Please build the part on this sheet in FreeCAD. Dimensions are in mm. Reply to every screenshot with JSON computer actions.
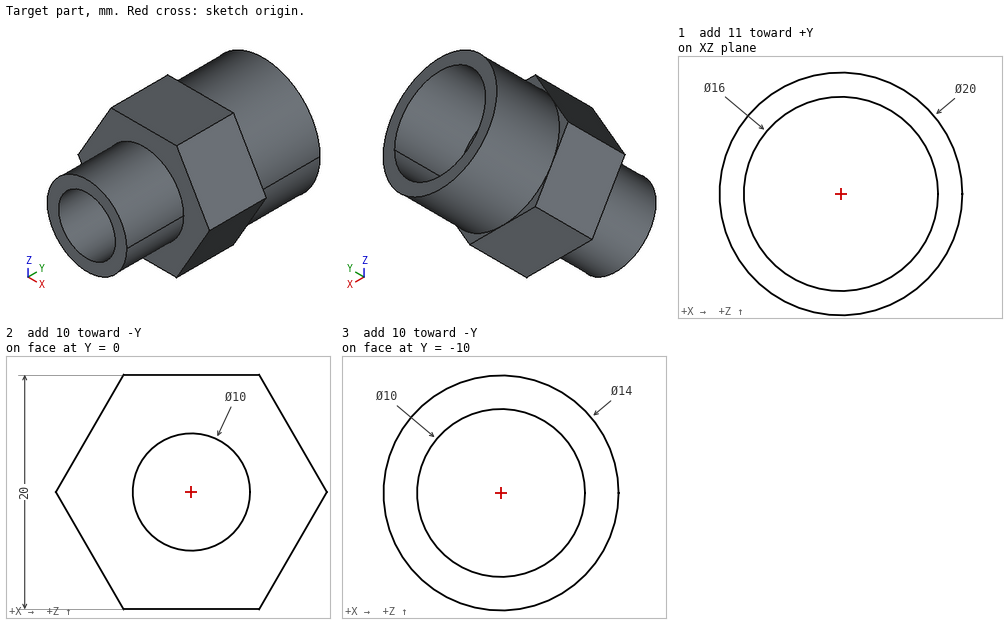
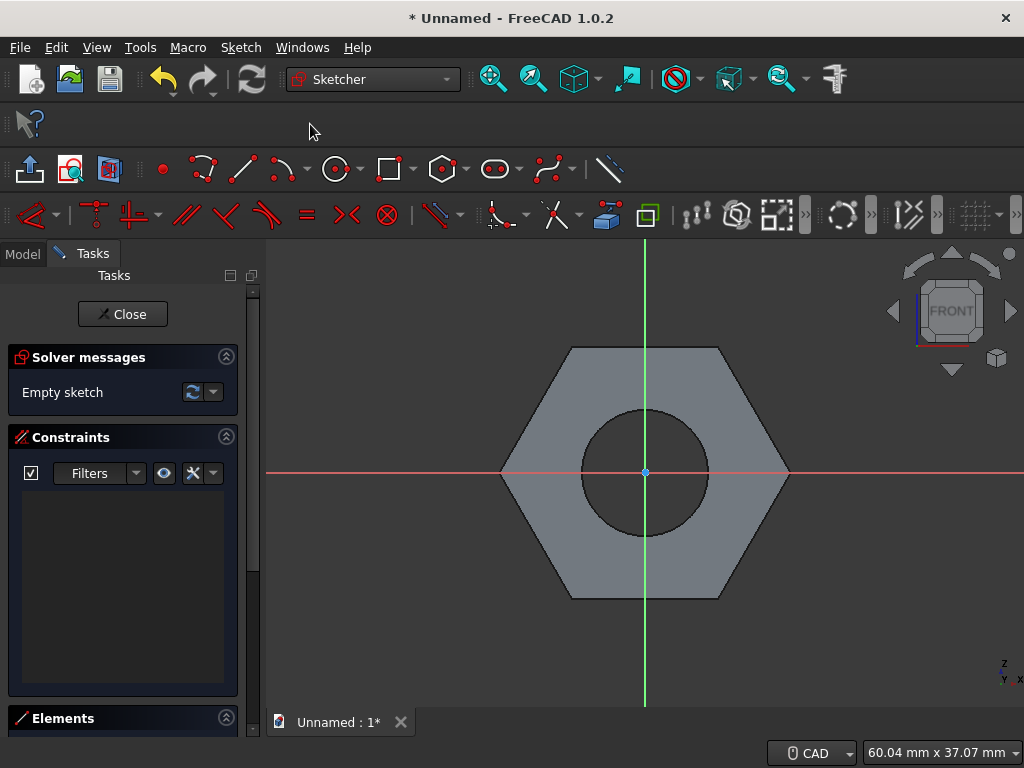
{"action": "scroll", "coordinate": [784, 473], "scroll_direction": "up", "scroll_amount": 2}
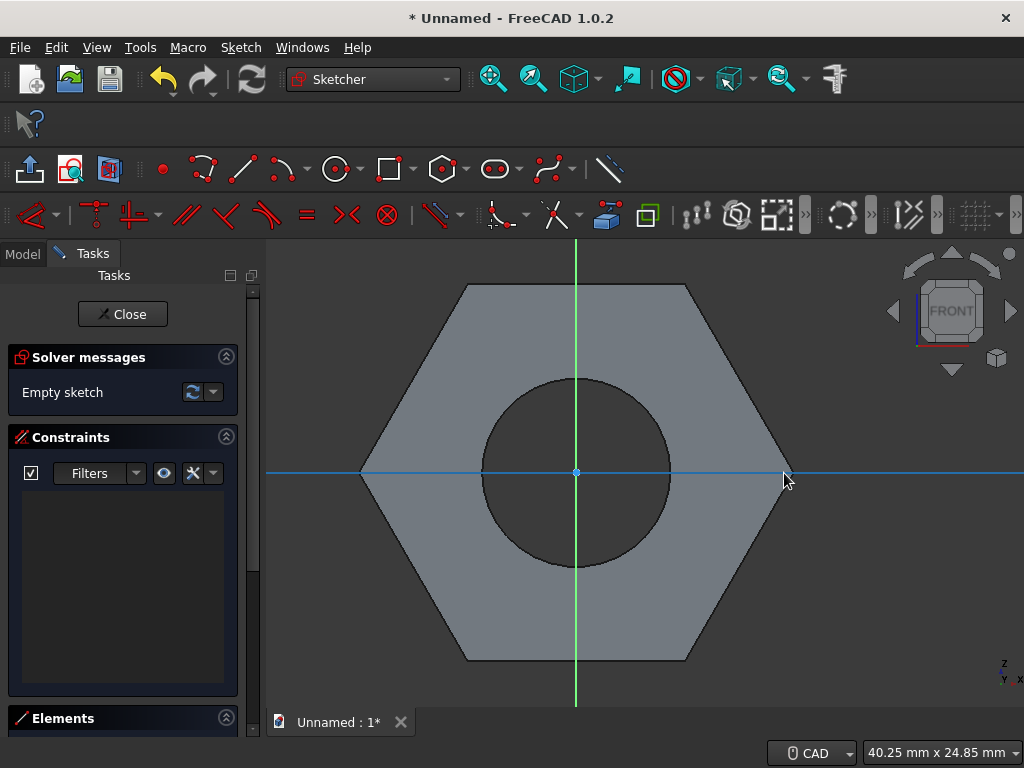
{"action": "left_click", "coordinate": [336, 170]}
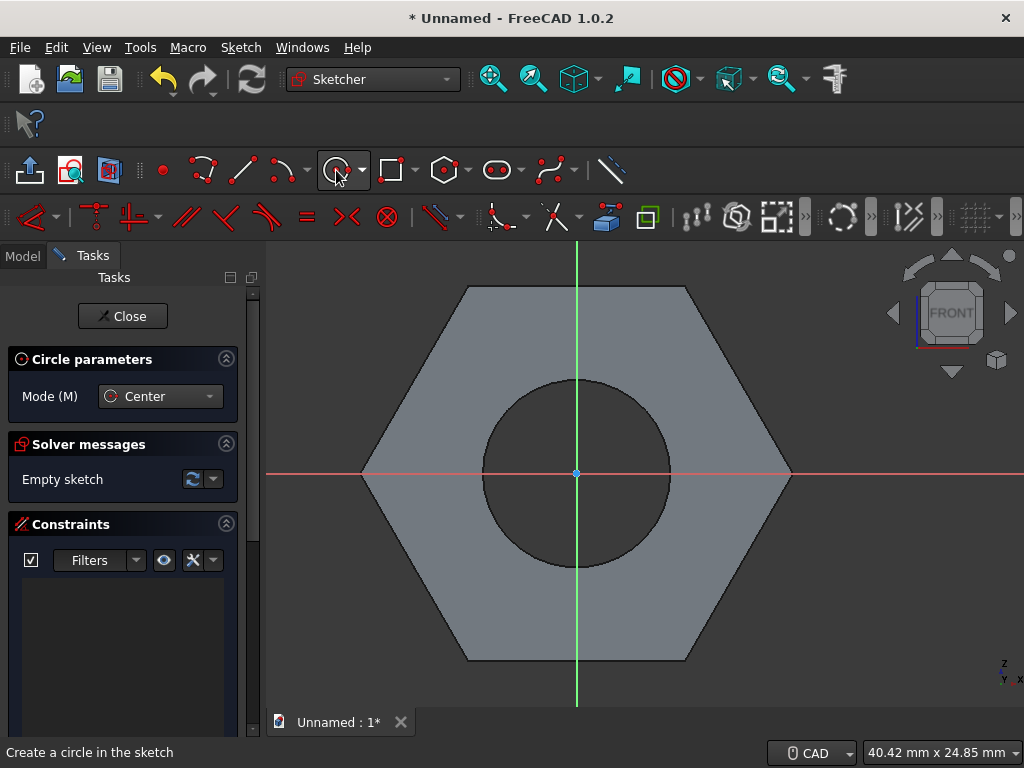
{"action": "left_click", "coordinate": [577, 474]}
{"action": "left_click", "coordinate": [669, 381]}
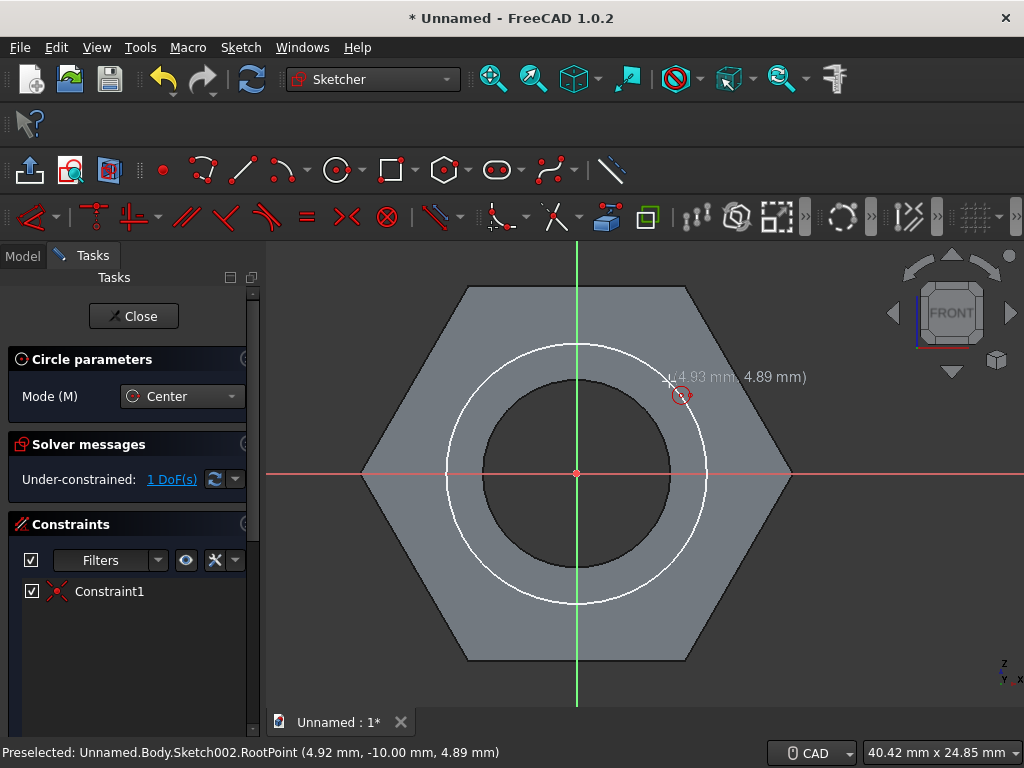
{"action": "left_click", "coordinate": [577, 474]}
{"action": "left_click", "coordinate": [643, 407]}
{"action": "key", "text": "Escape"}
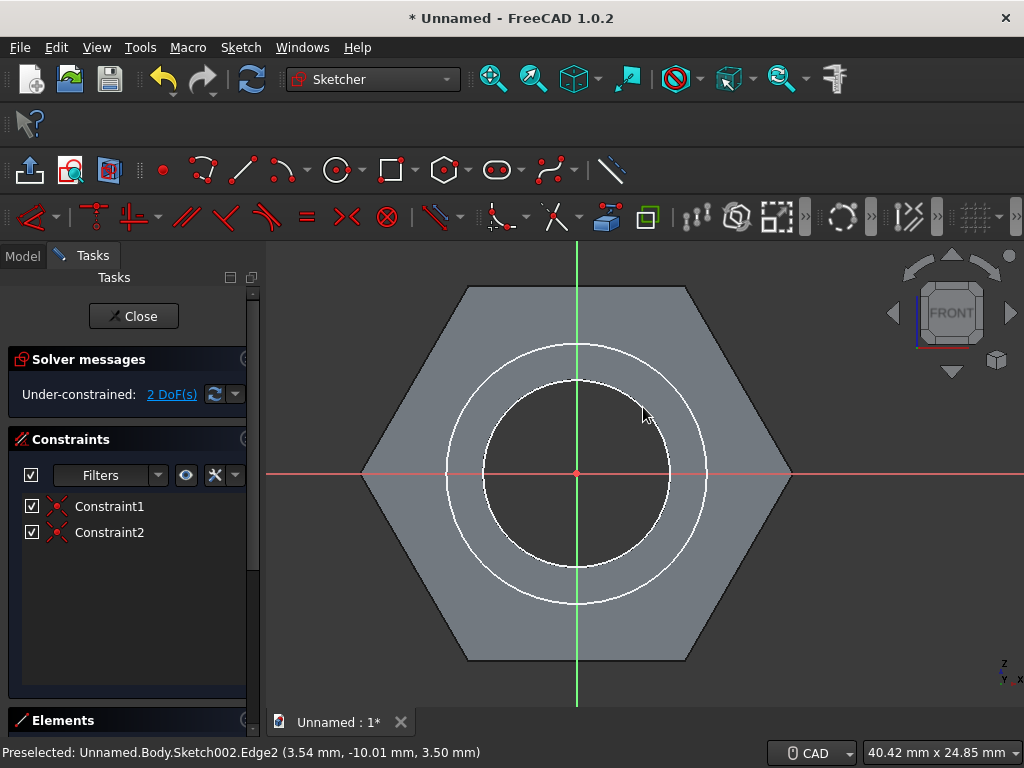
{"action": "left_click", "coordinate": [32, 218]}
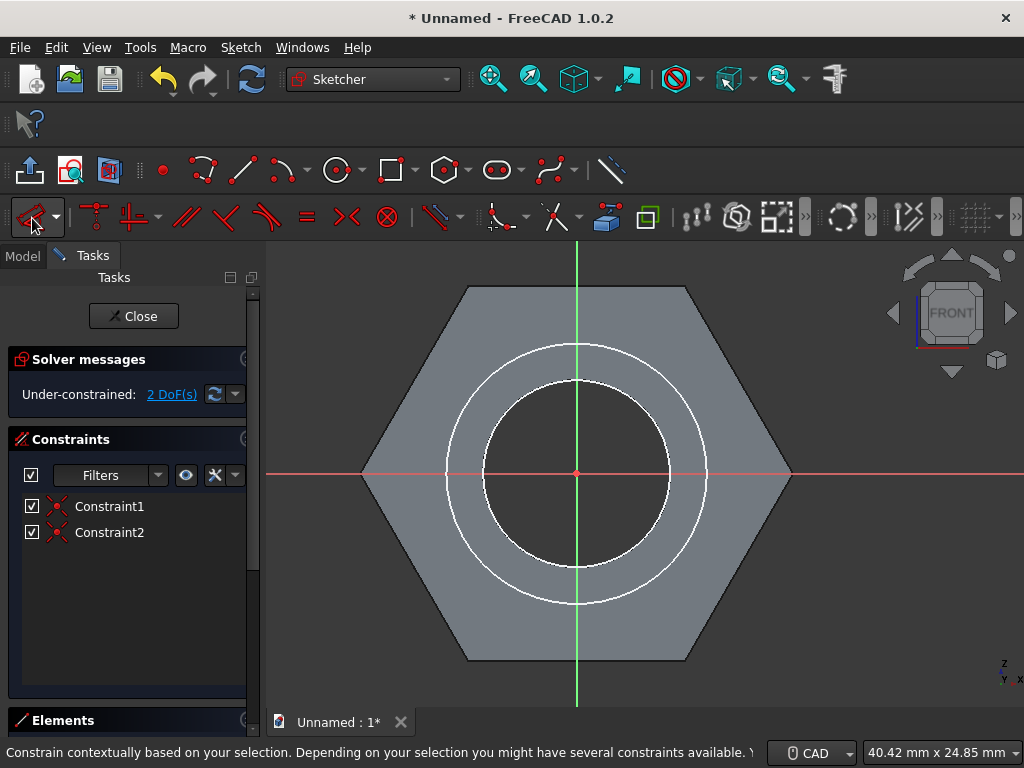
{"action": "left_click", "coordinate": [668, 381]}
{"action": "left_click", "coordinate": [690, 358]}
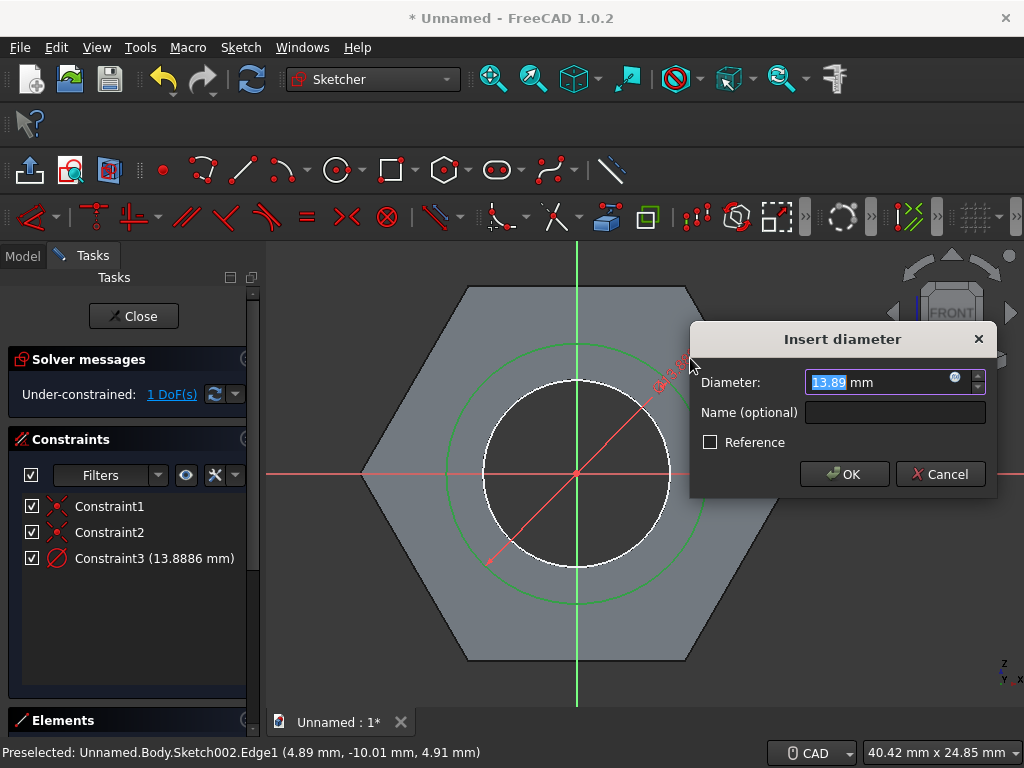
{"action": "type", "text": "14"}
{"action": "key", "text": "Return"}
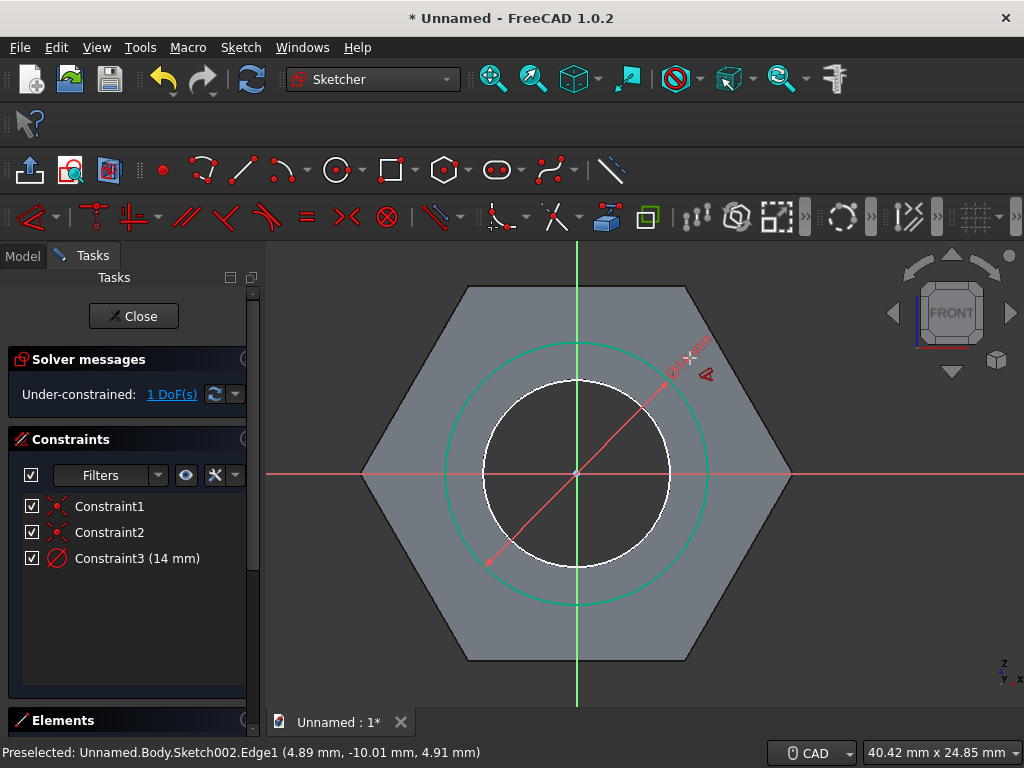
{"action": "left_click", "coordinate": [642, 407]}
{"action": "left_click", "coordinate": [719, 431]}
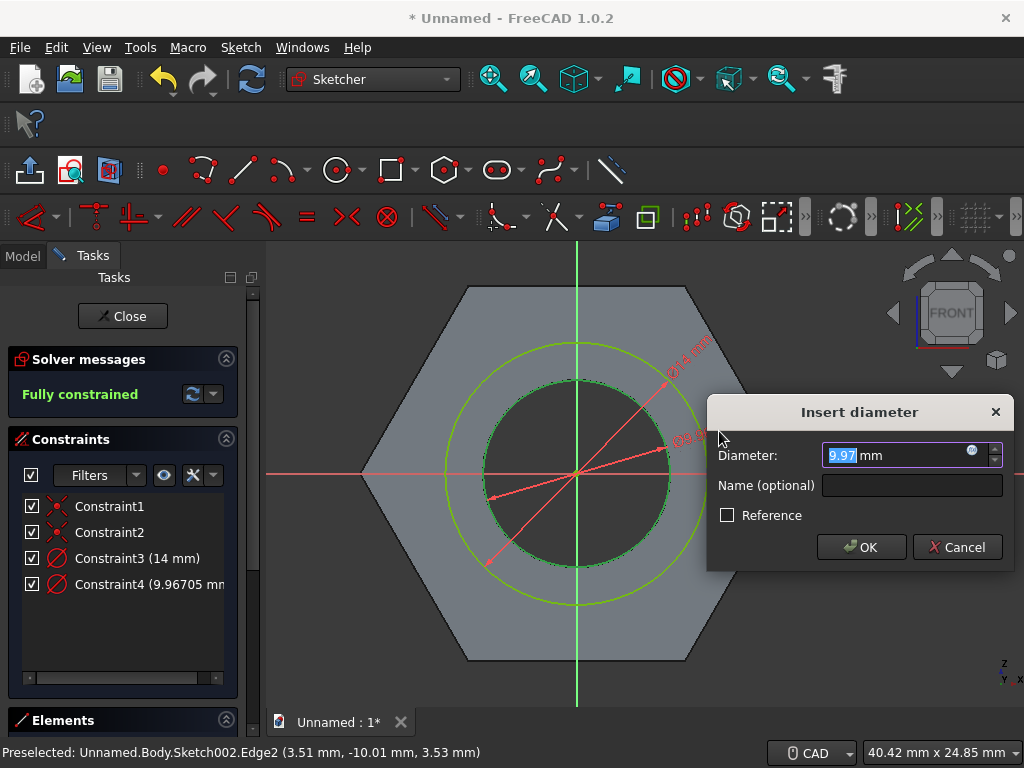
{"action": "type", "text": "10"}
{"action": "key", "text": "Return"}
{"action": "key", "text": "Escape"}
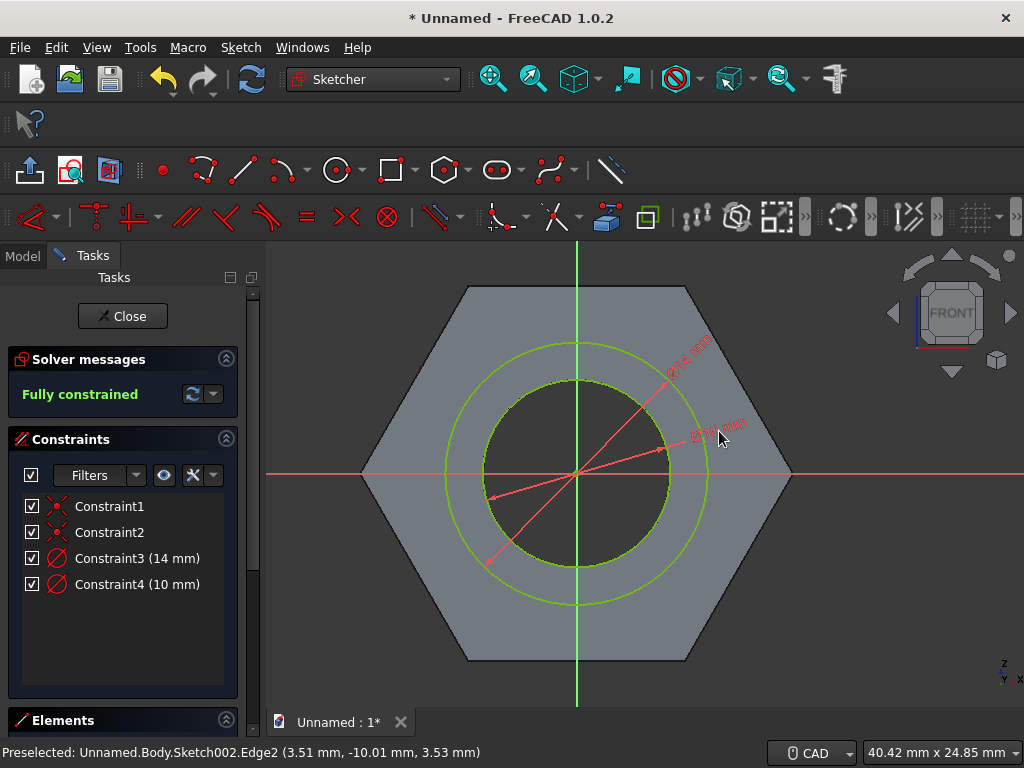
{"action": "left_click", "coordinate": [123, 316]}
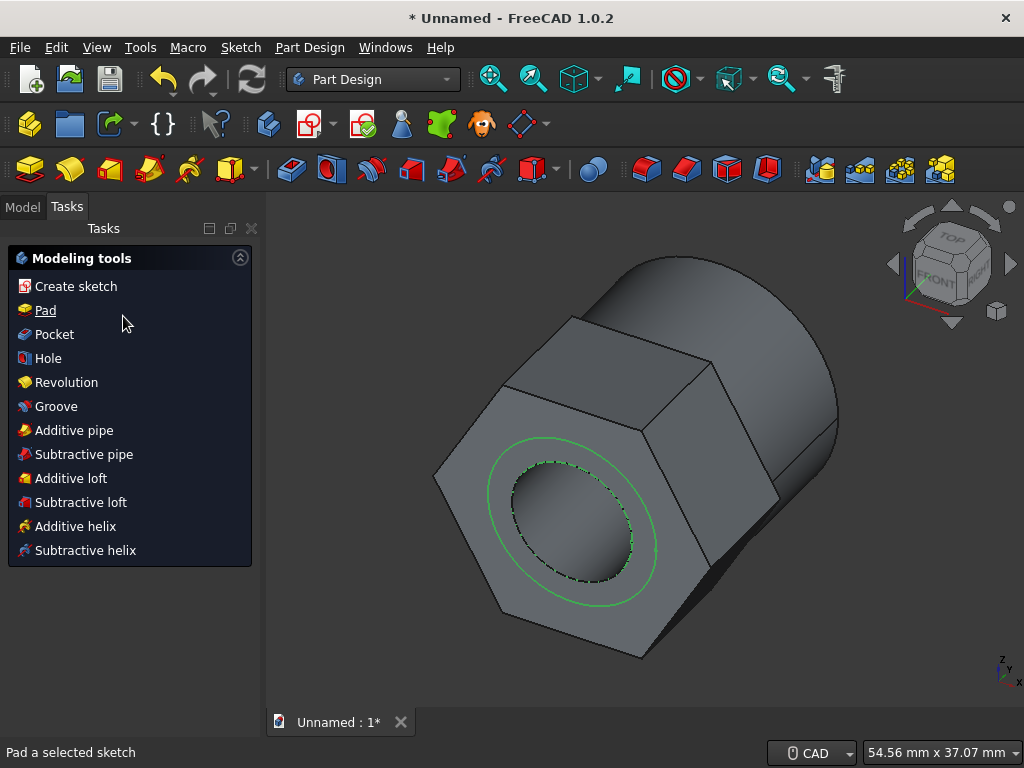
{"action": "left_click", "coordinate": [30, 170]}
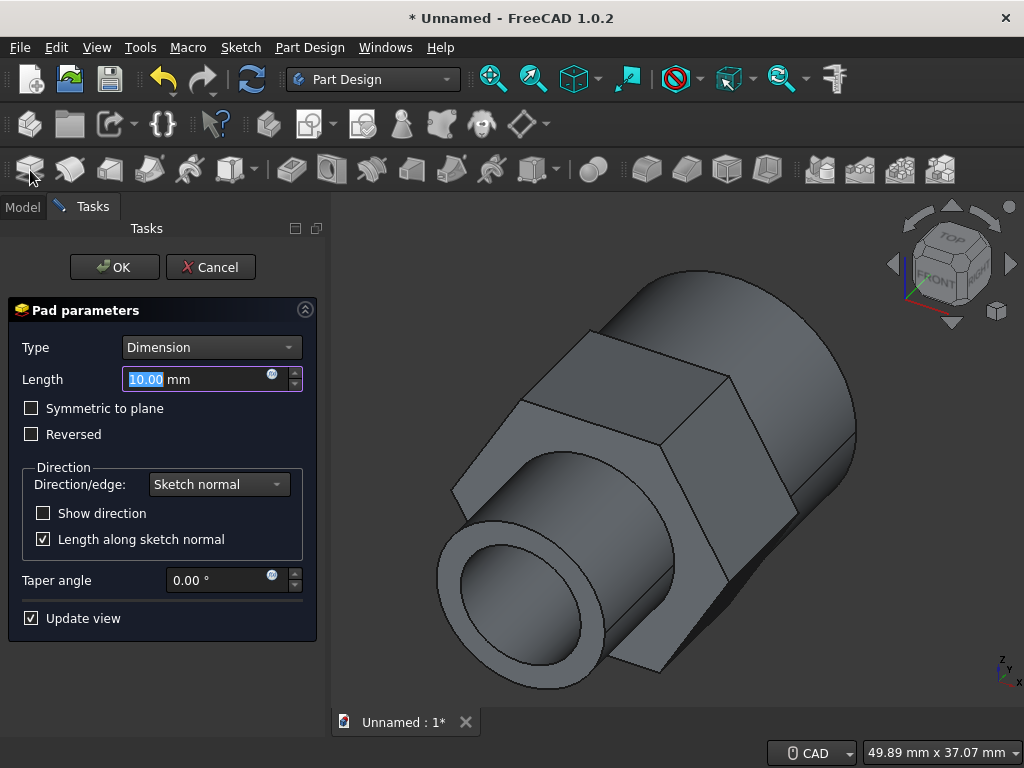
{"action": "type", "text": "10"}
{"action": "key", "text": "Tab"}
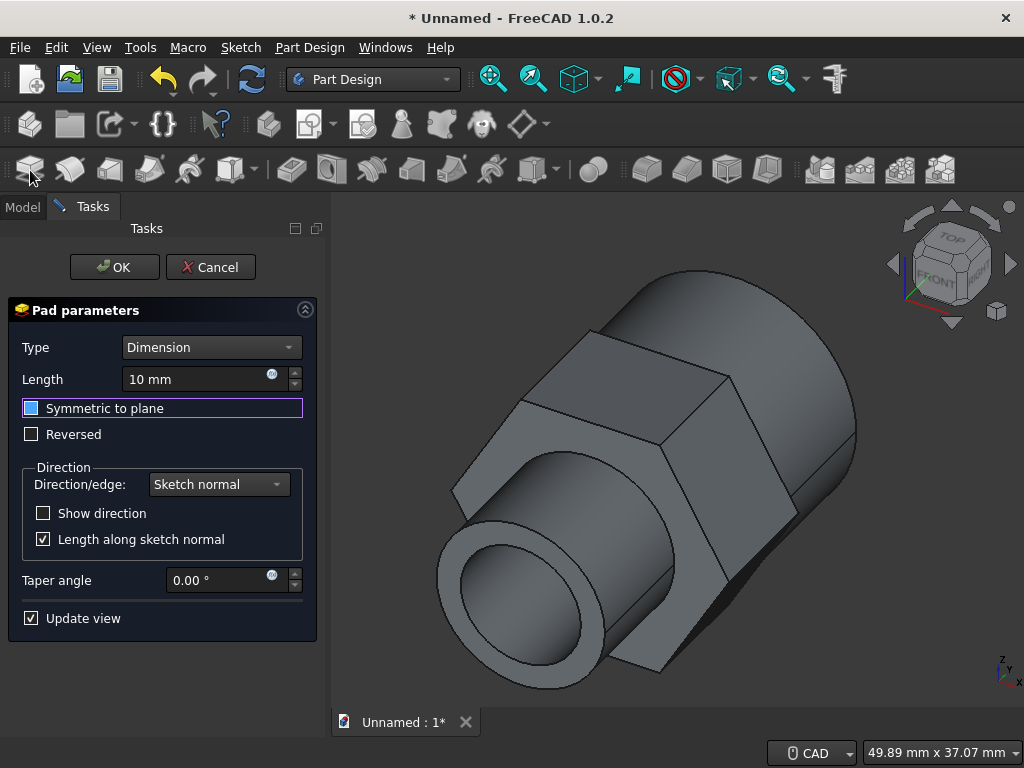
{"action": "left_click", "coordinate": [115, 267]}